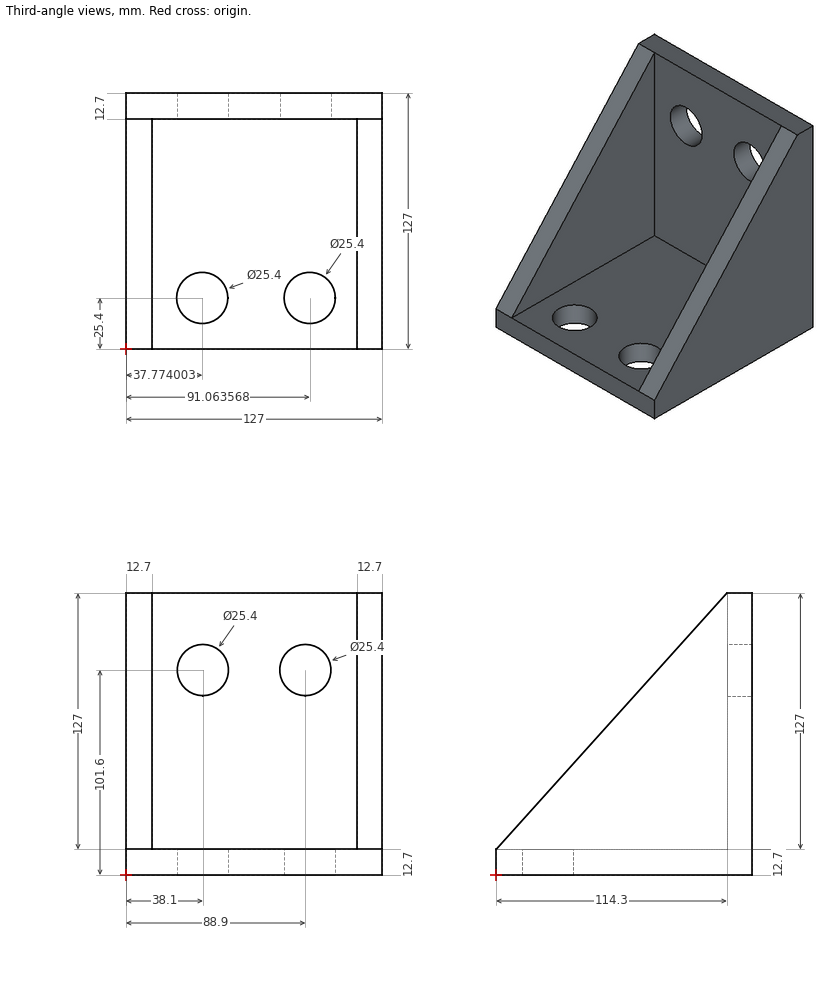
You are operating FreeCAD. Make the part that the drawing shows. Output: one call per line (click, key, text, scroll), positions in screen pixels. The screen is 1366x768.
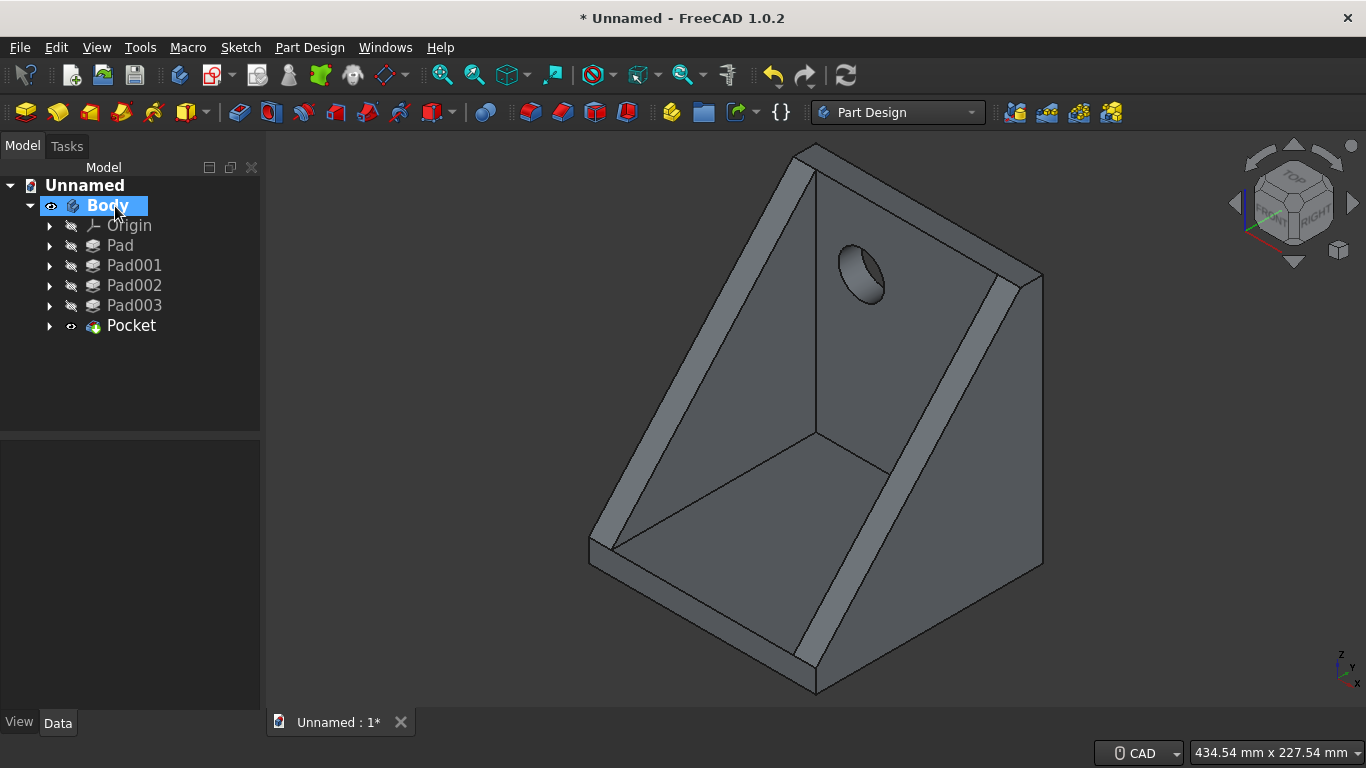
click(907, 390)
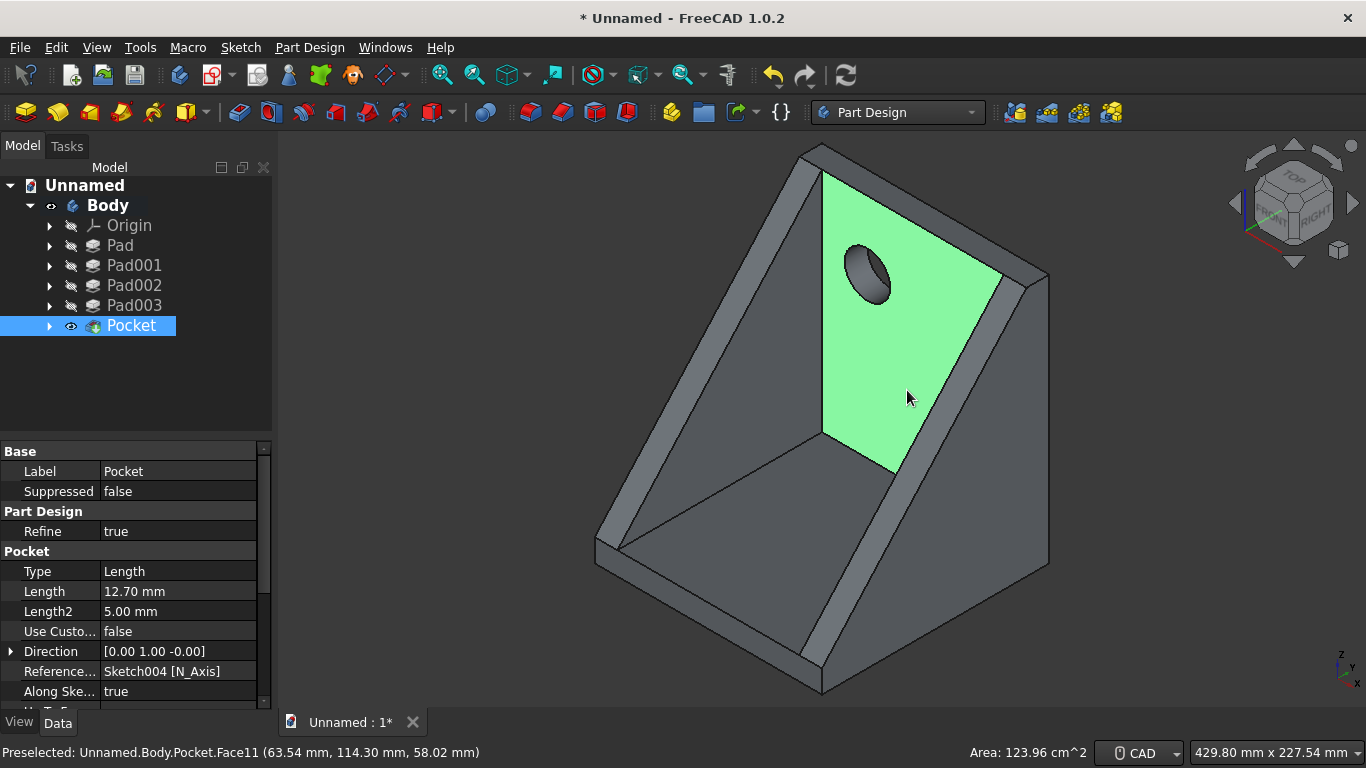
click(212, 76)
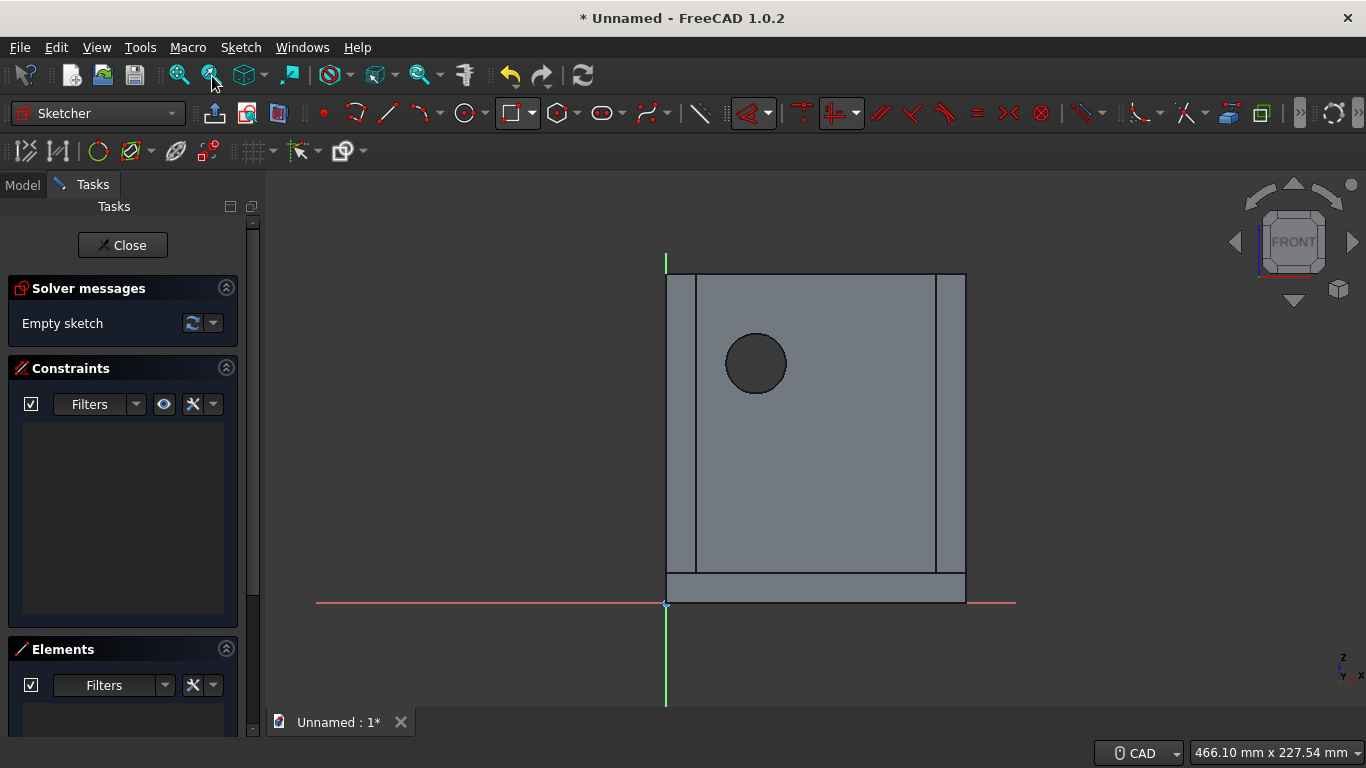
click(280, 114)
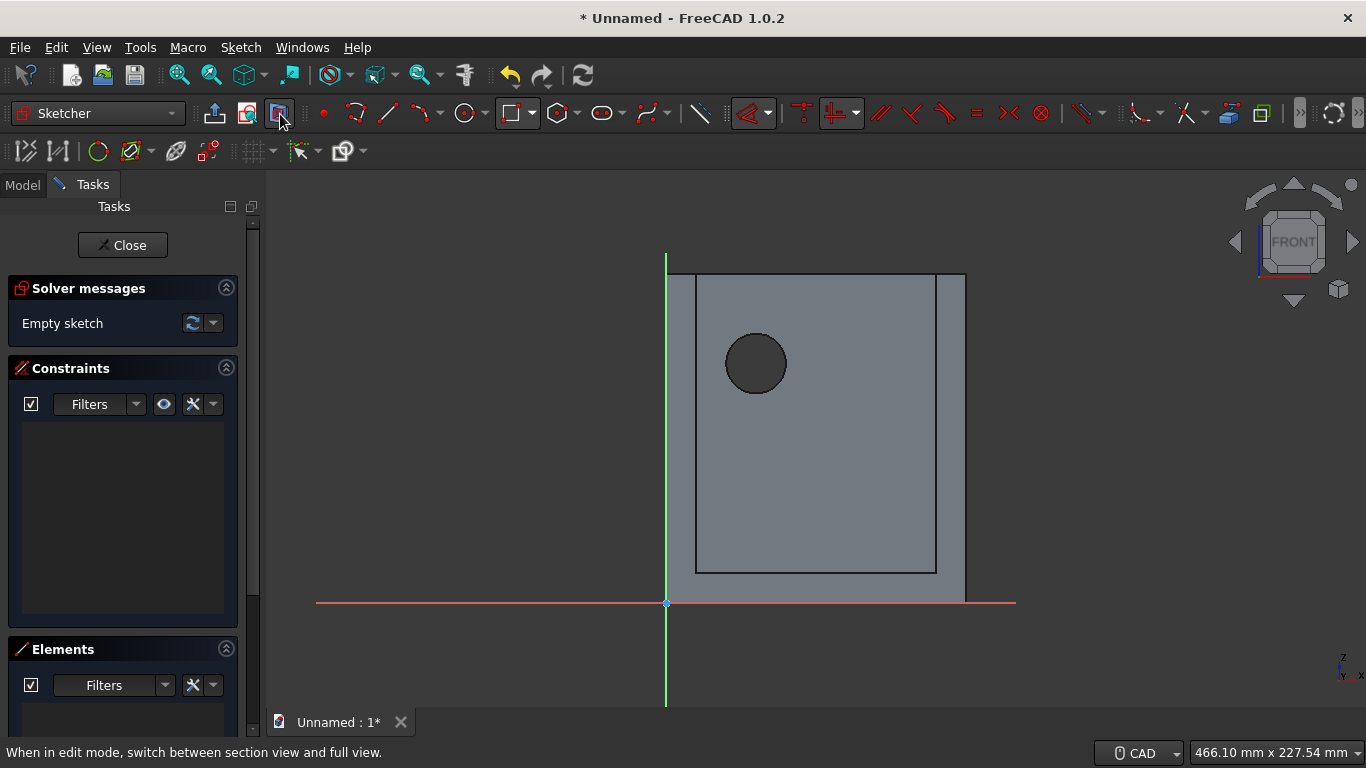
scroll(901, 349, up, 9)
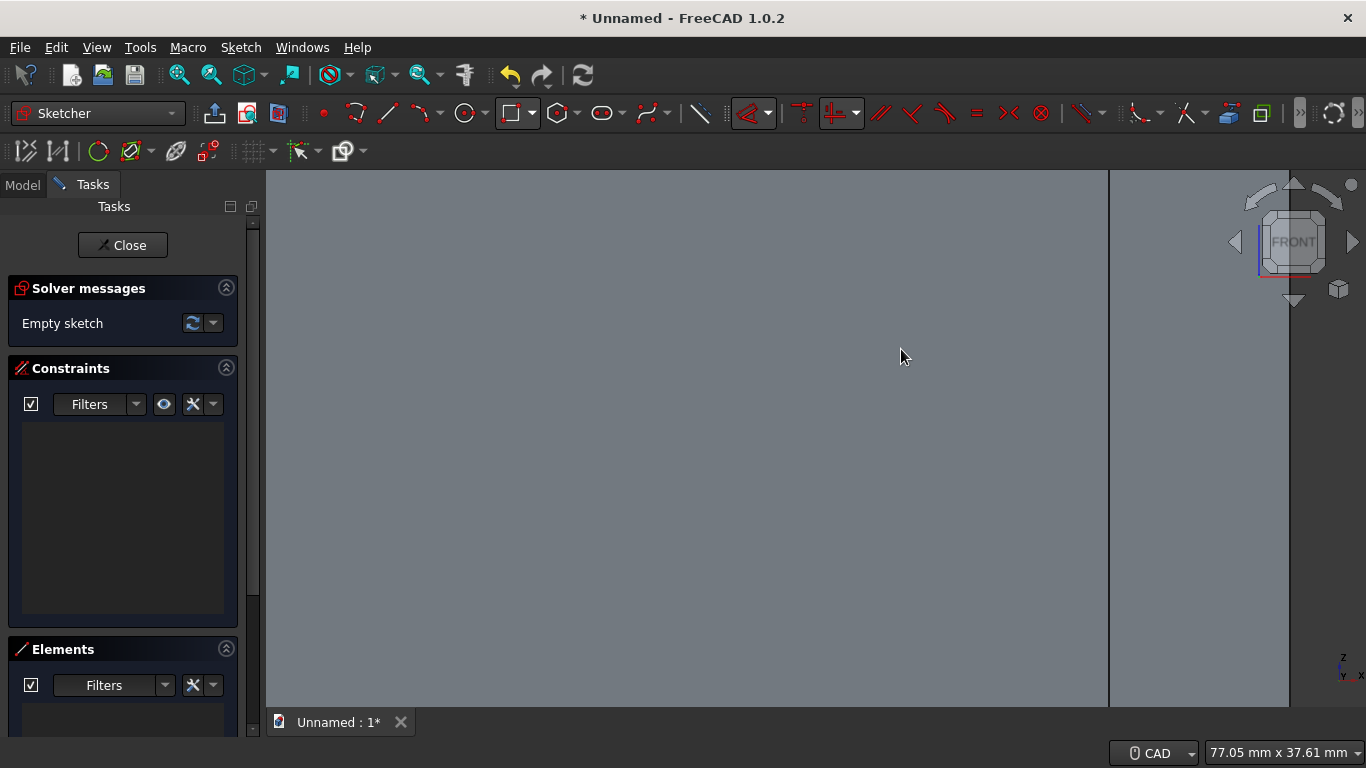
key(g)
key(c)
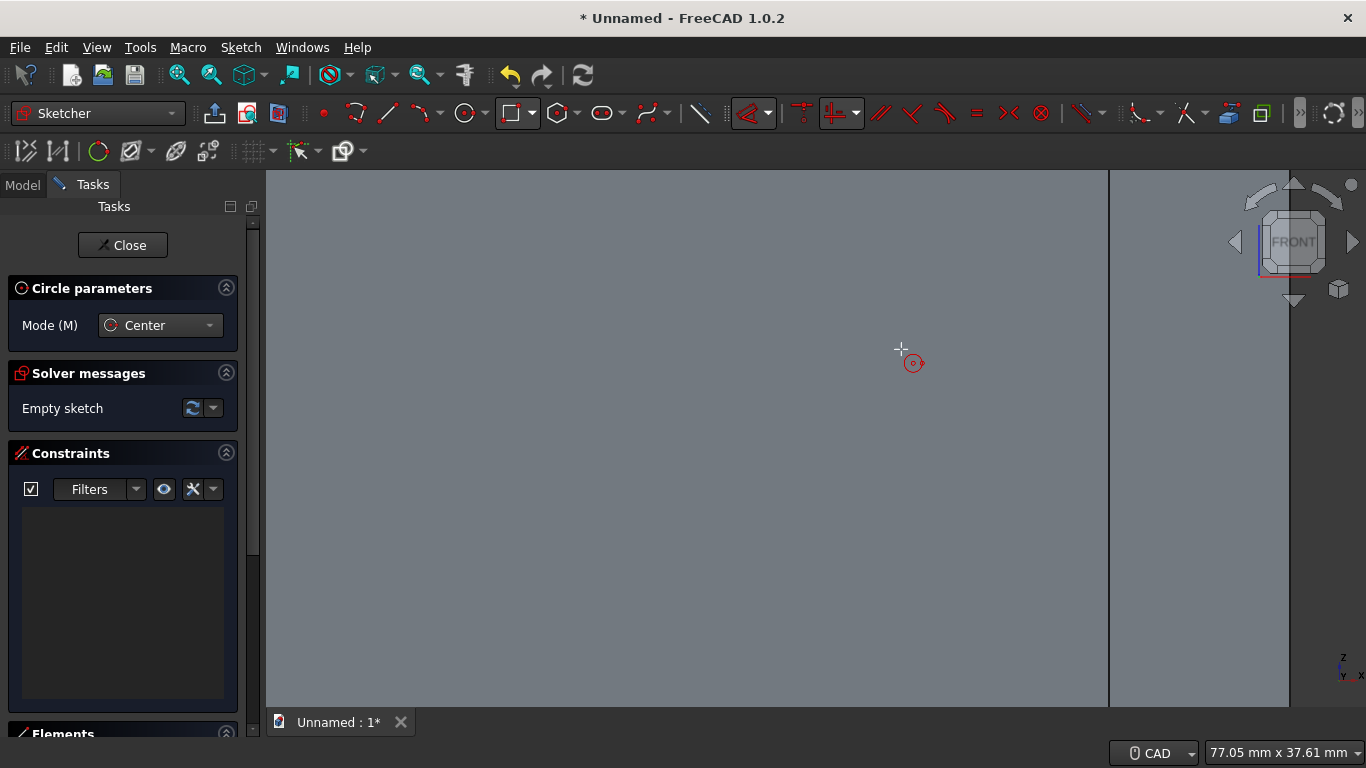
click(747, 435)
click(875, 307)
key(Escape)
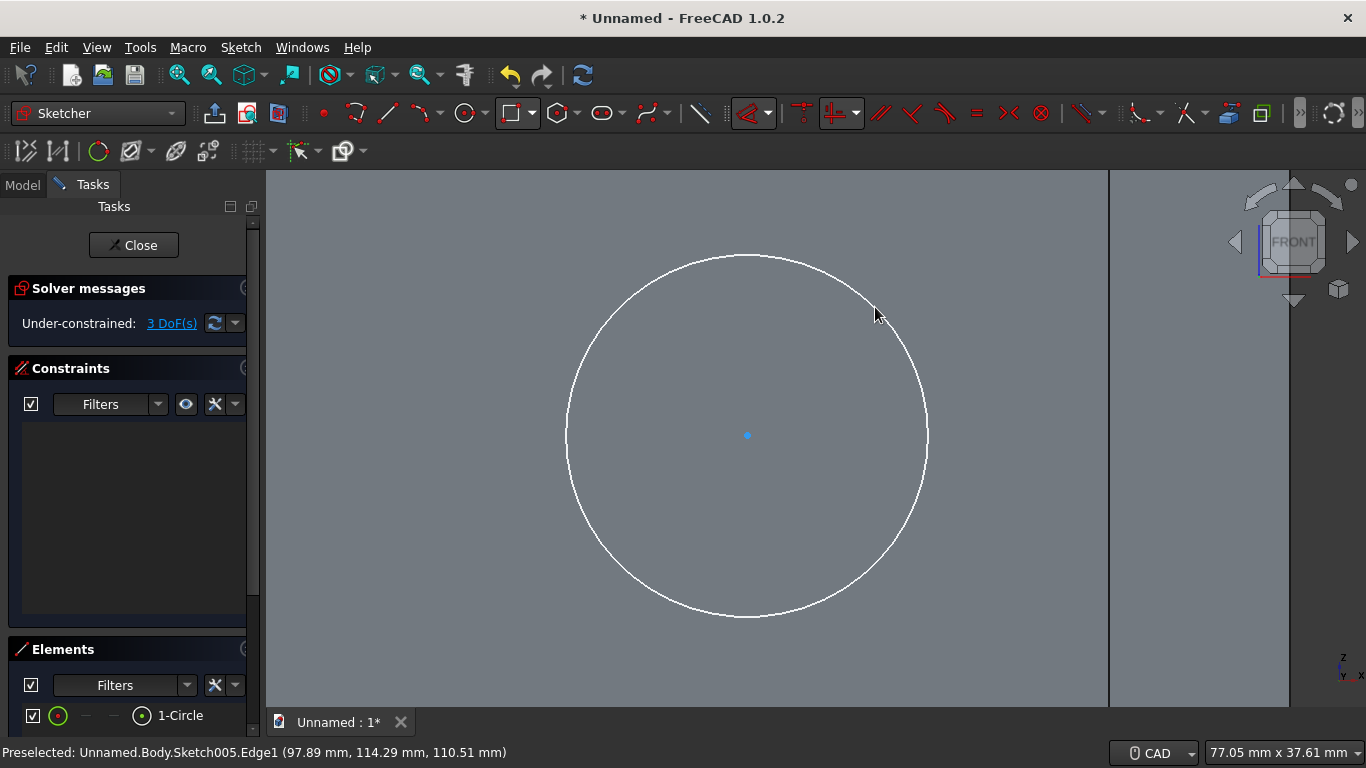
click(875, 308)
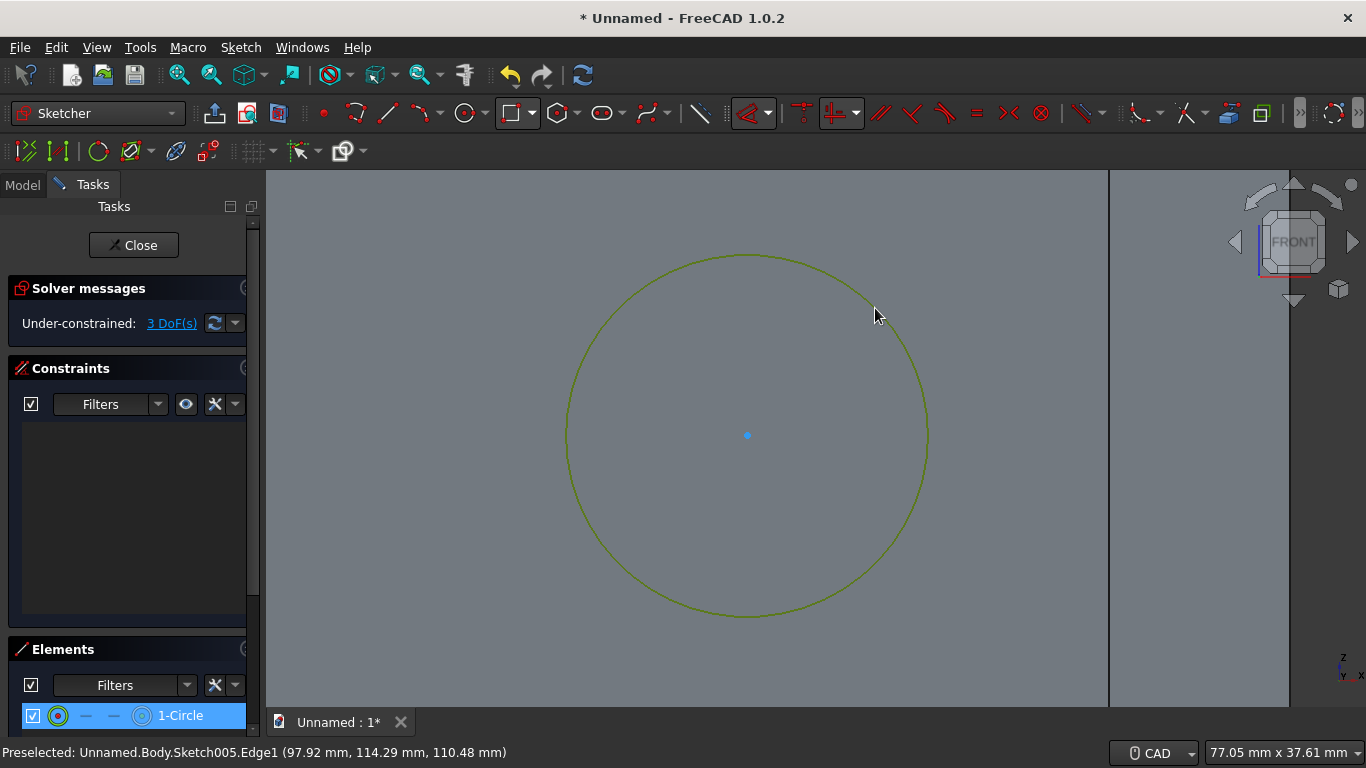
key(k)
key(o)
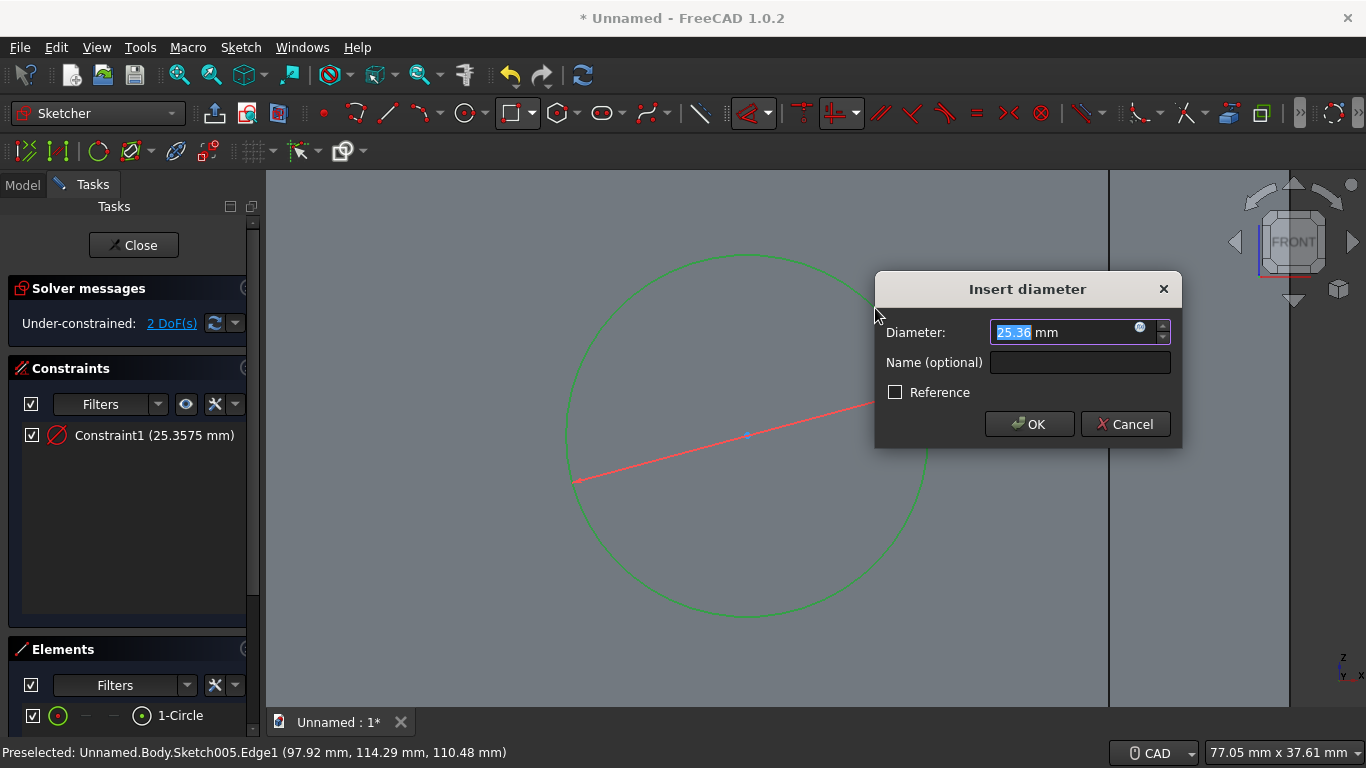
text(25.4)
key(Return)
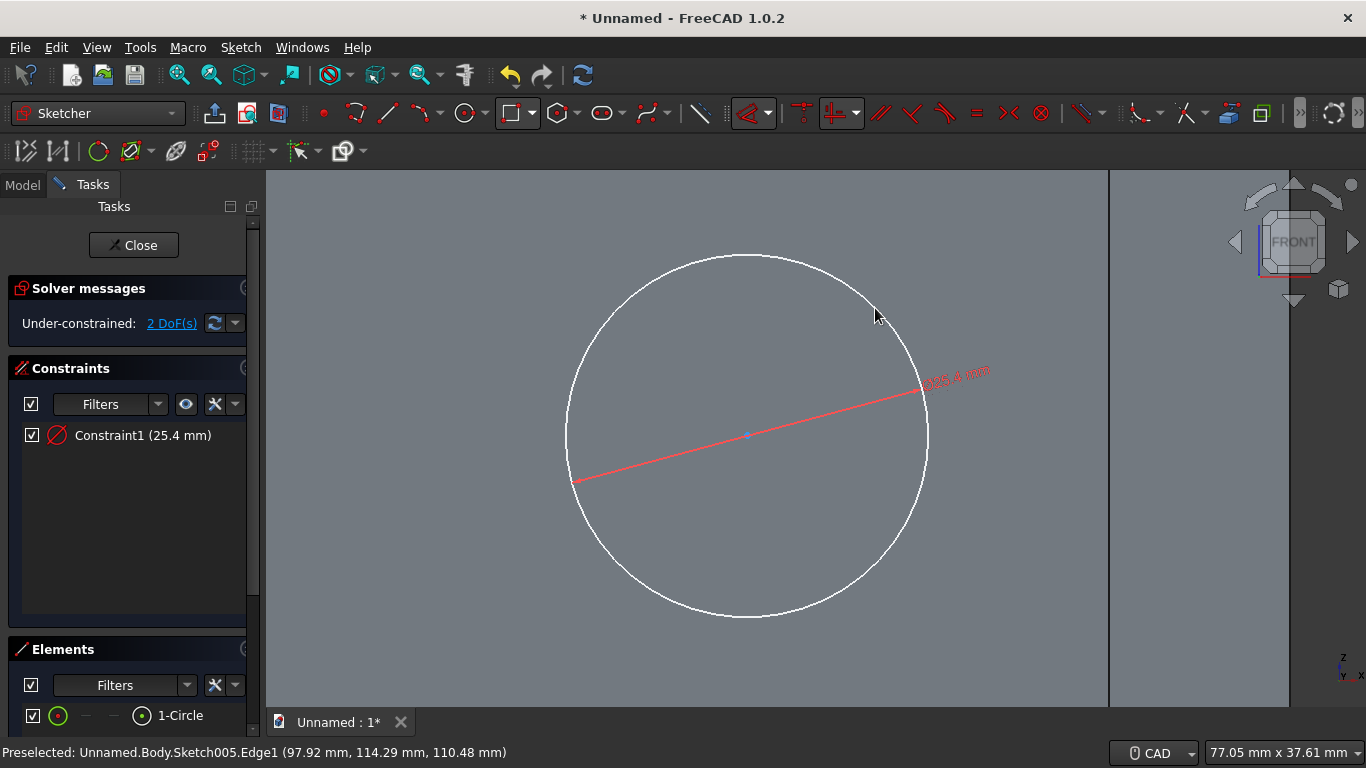
click(747, 436)